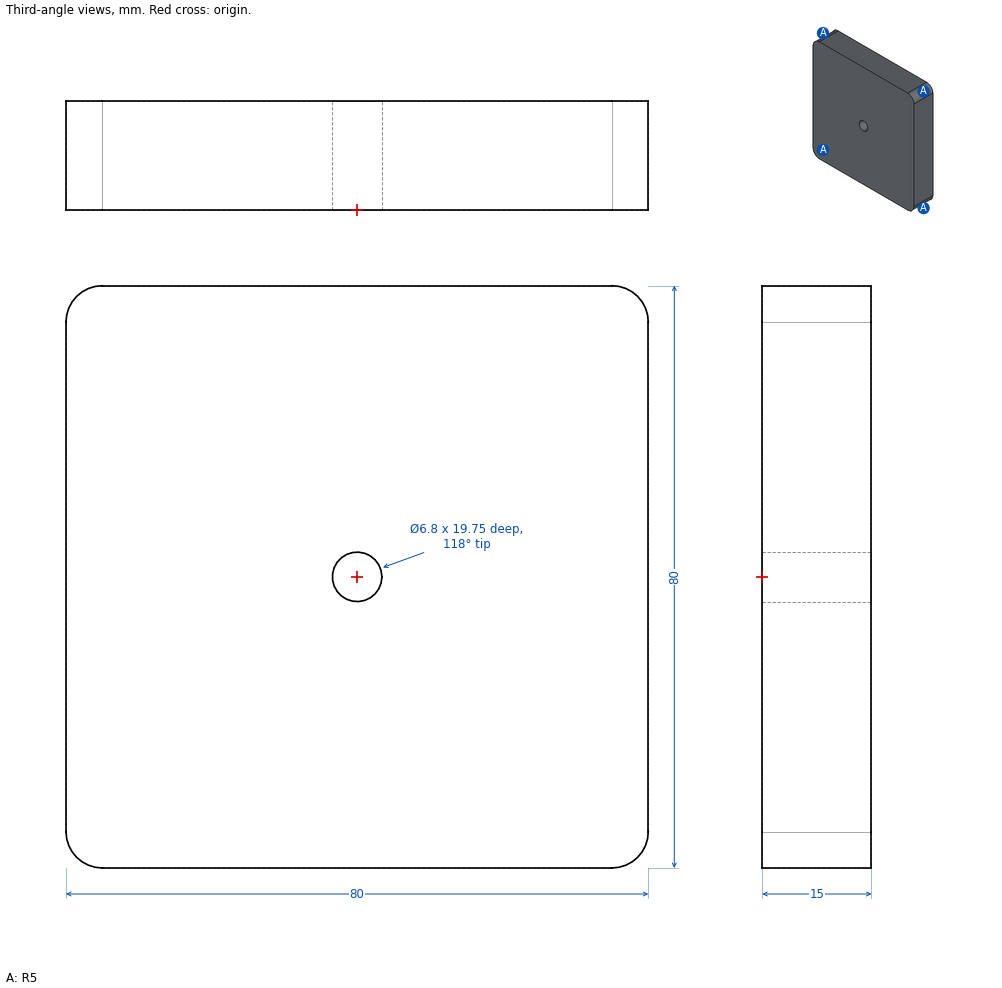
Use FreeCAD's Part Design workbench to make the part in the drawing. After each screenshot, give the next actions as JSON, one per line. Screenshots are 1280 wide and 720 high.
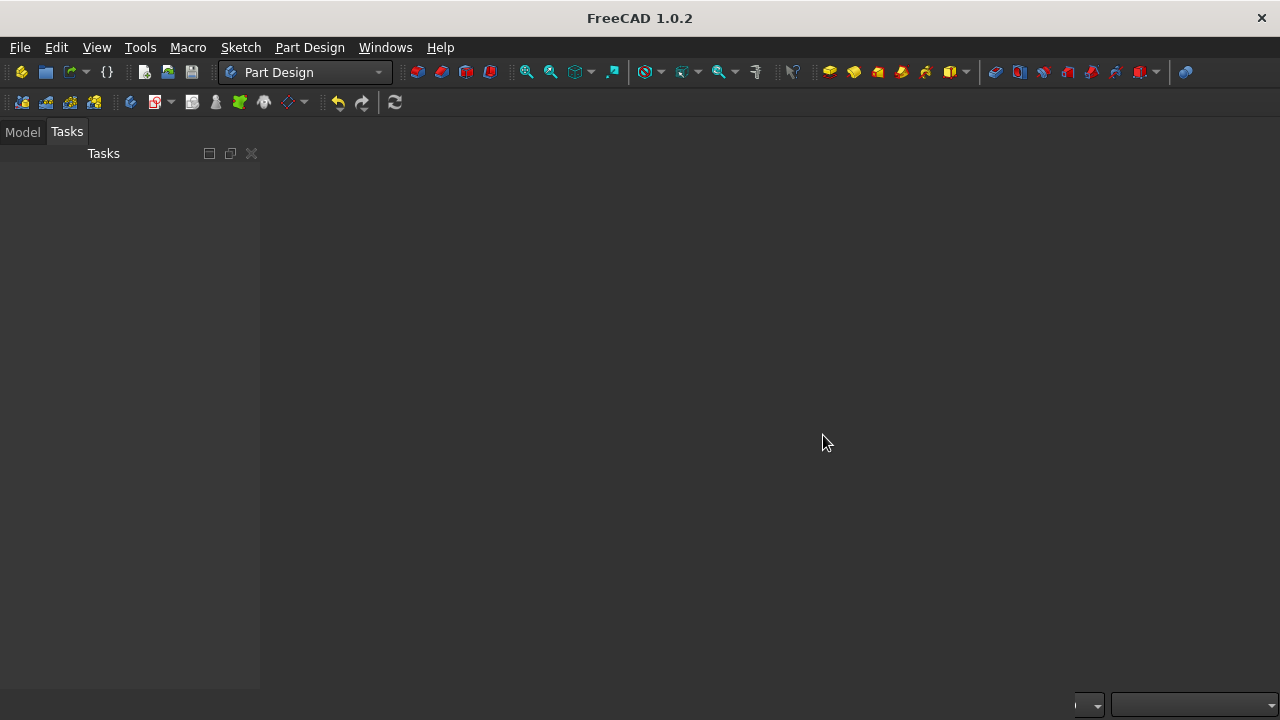
{"action": "key", "text": "ctrl+n"}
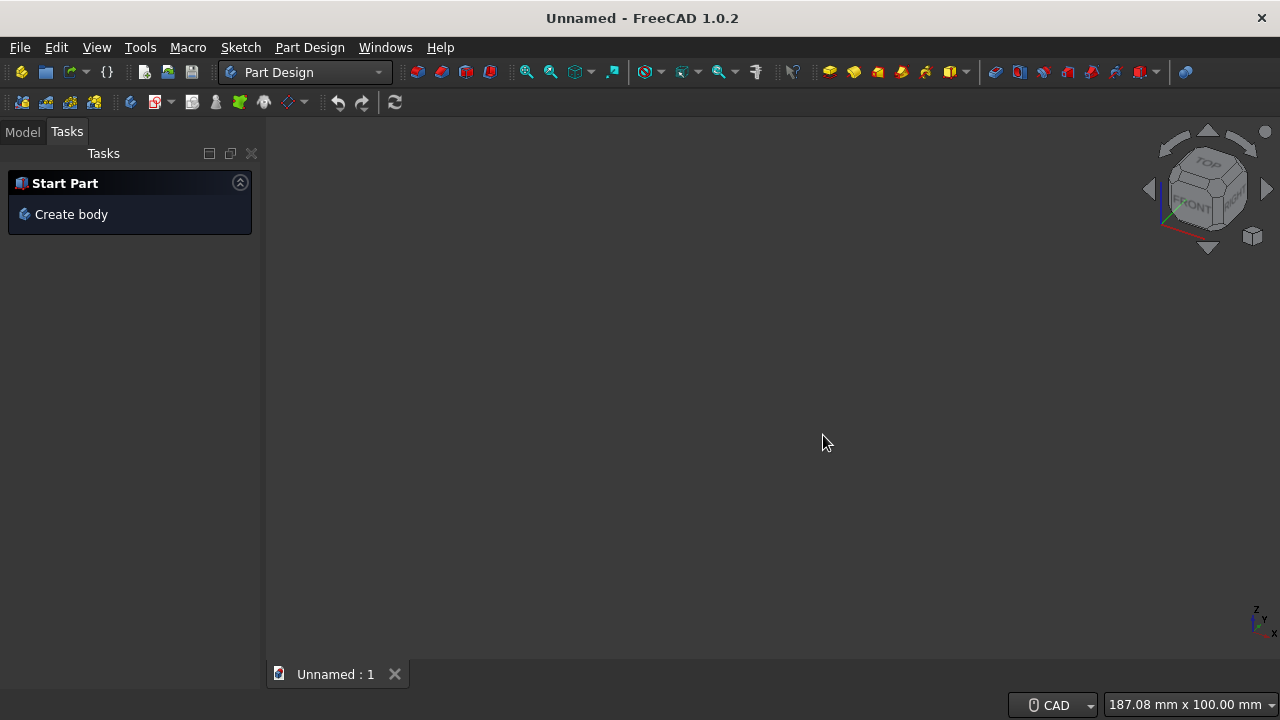
{"action": "left_click", "coordinate": [156, 102]}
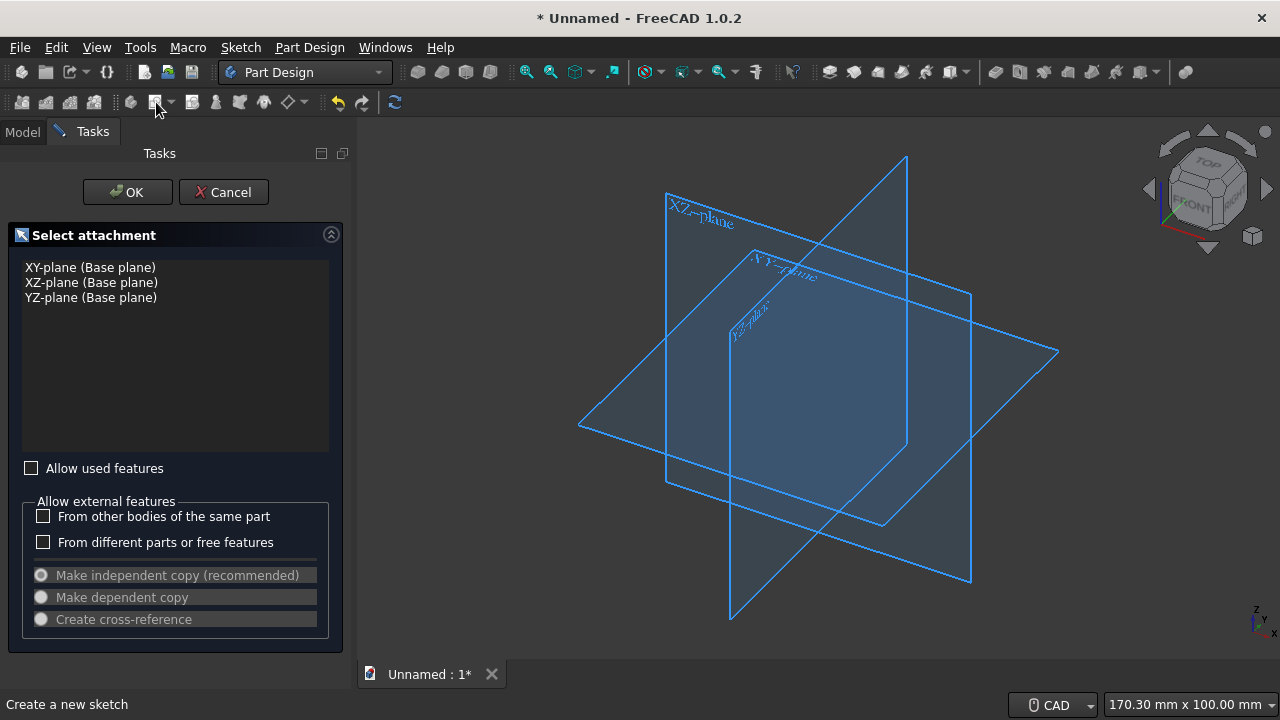
{"action": "left_click", "coordinate": [82, 282]}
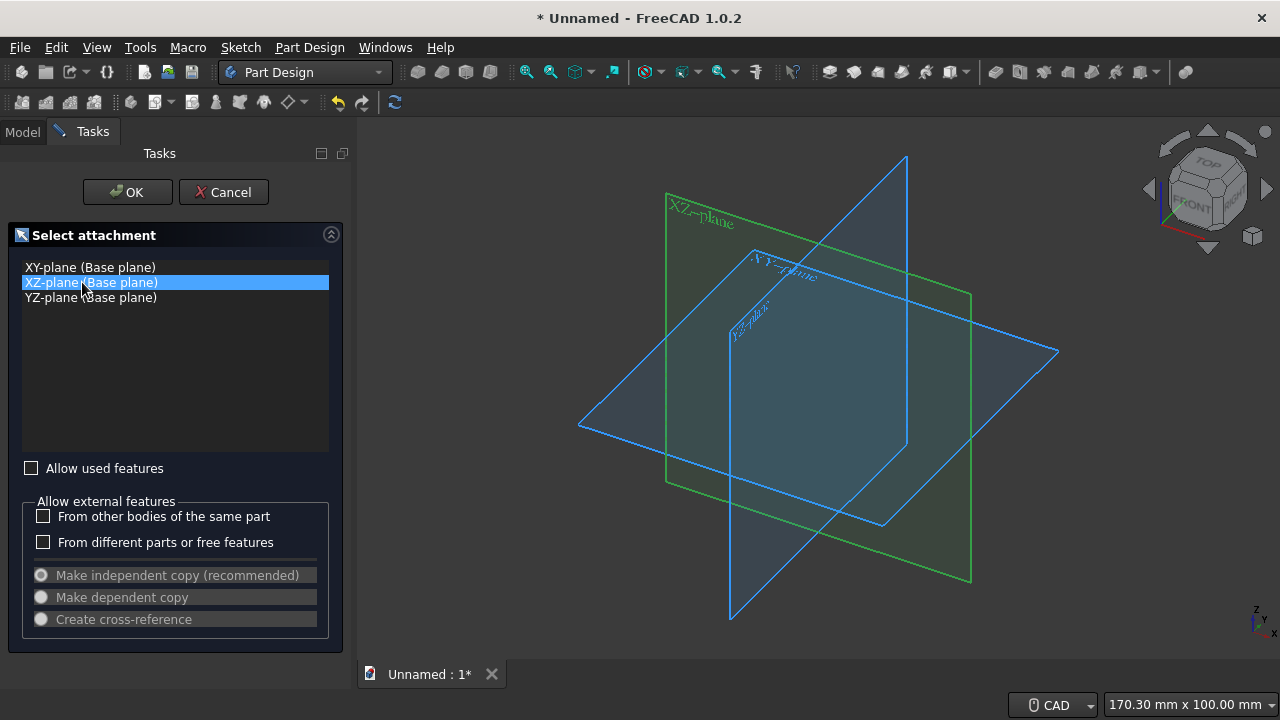
{"action": "left_click", "coordinate": [128, 192]}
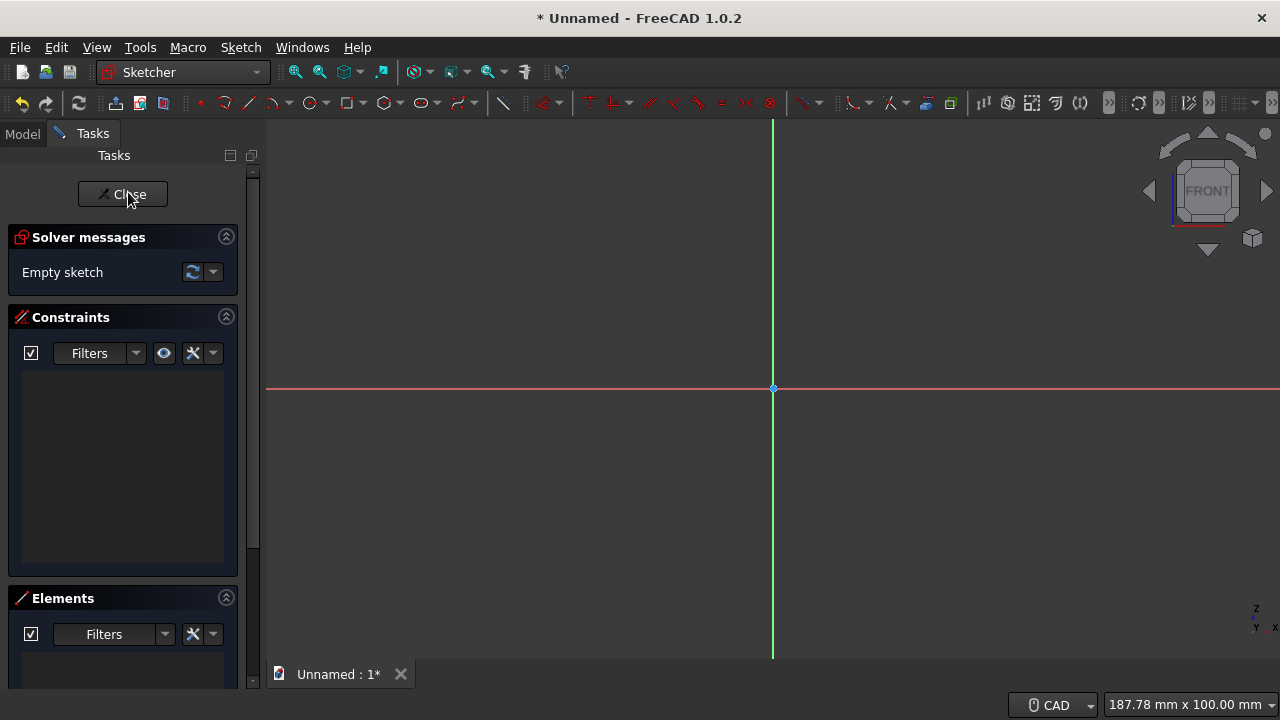
{"action": "key", "text": "g v"}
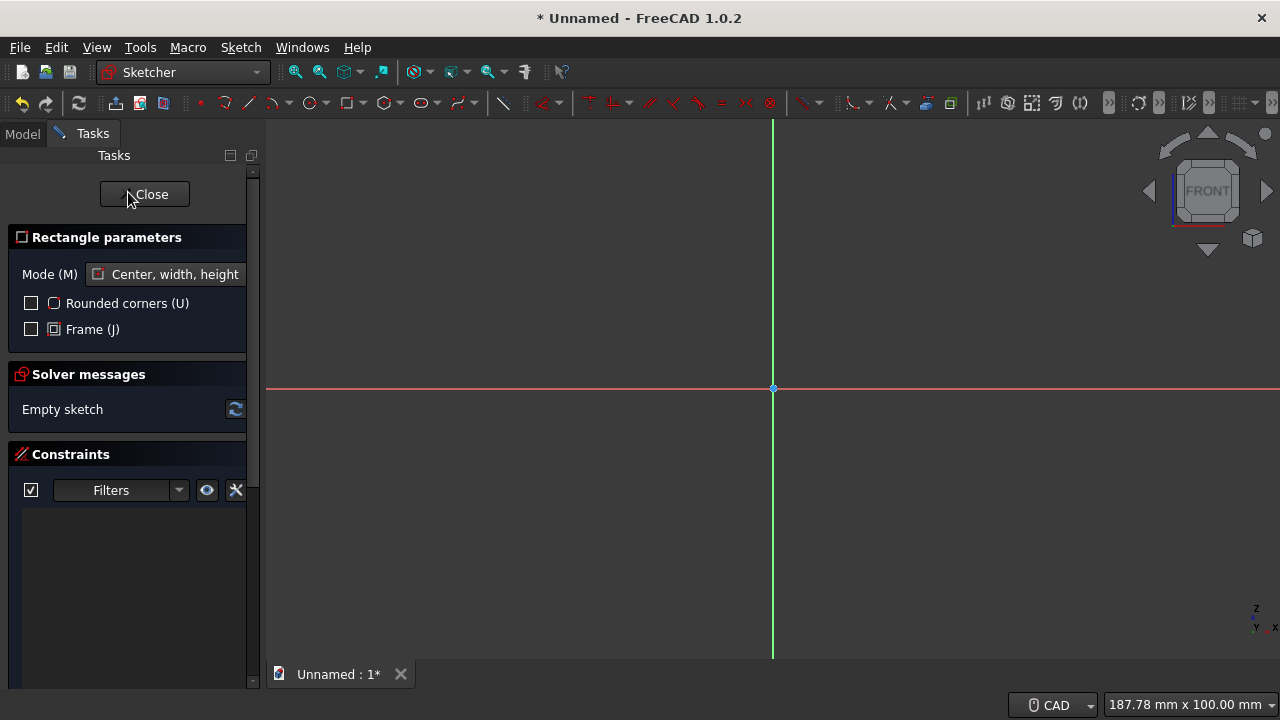
{"action": "left_click", "coordinate": [773, 389]}
{"action": "mouse_move", "coordinate": [989, 173]}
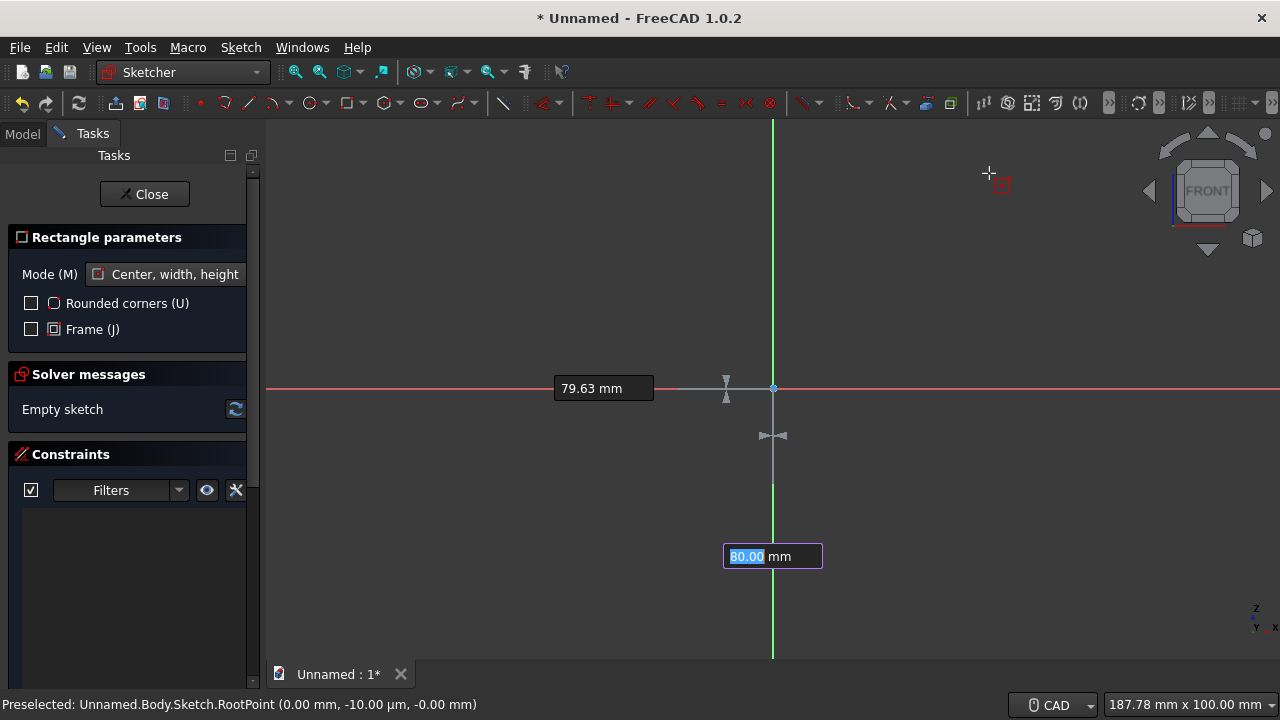
{"action": "type", "text": "80"}
{"action": "key", "text": "Tab"}
{"action": "type", "text": "80"}
{"action": "key", "text": "Return"}
{"action": "key", "text": "Escape"}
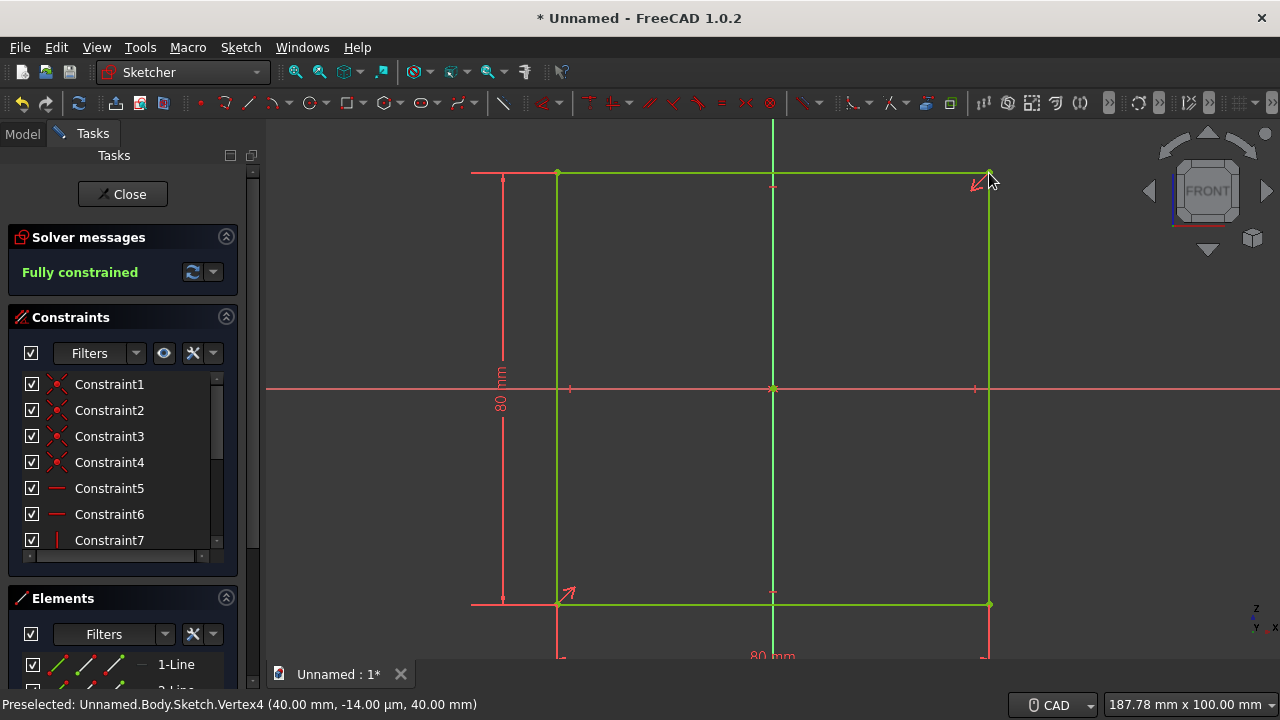
{"action": "left_click", "coordinate": [123, 194]}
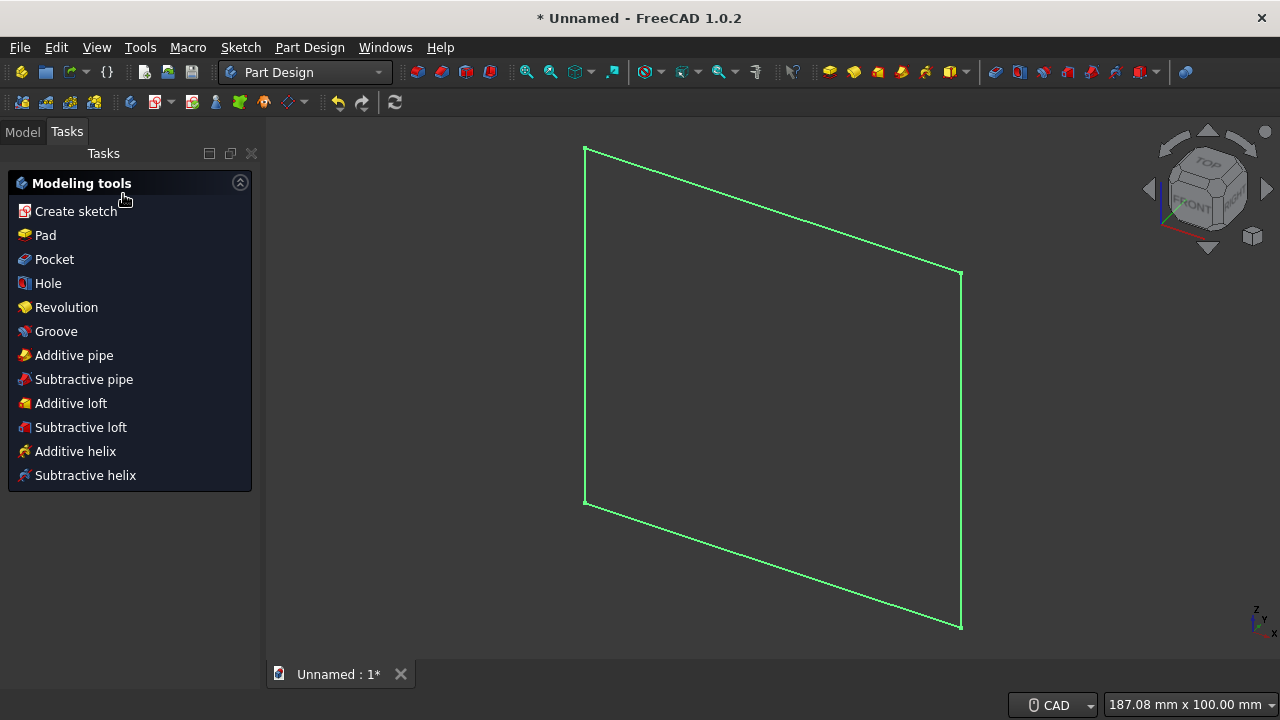
{"action": "left_click", "coordinate": [830, 72]}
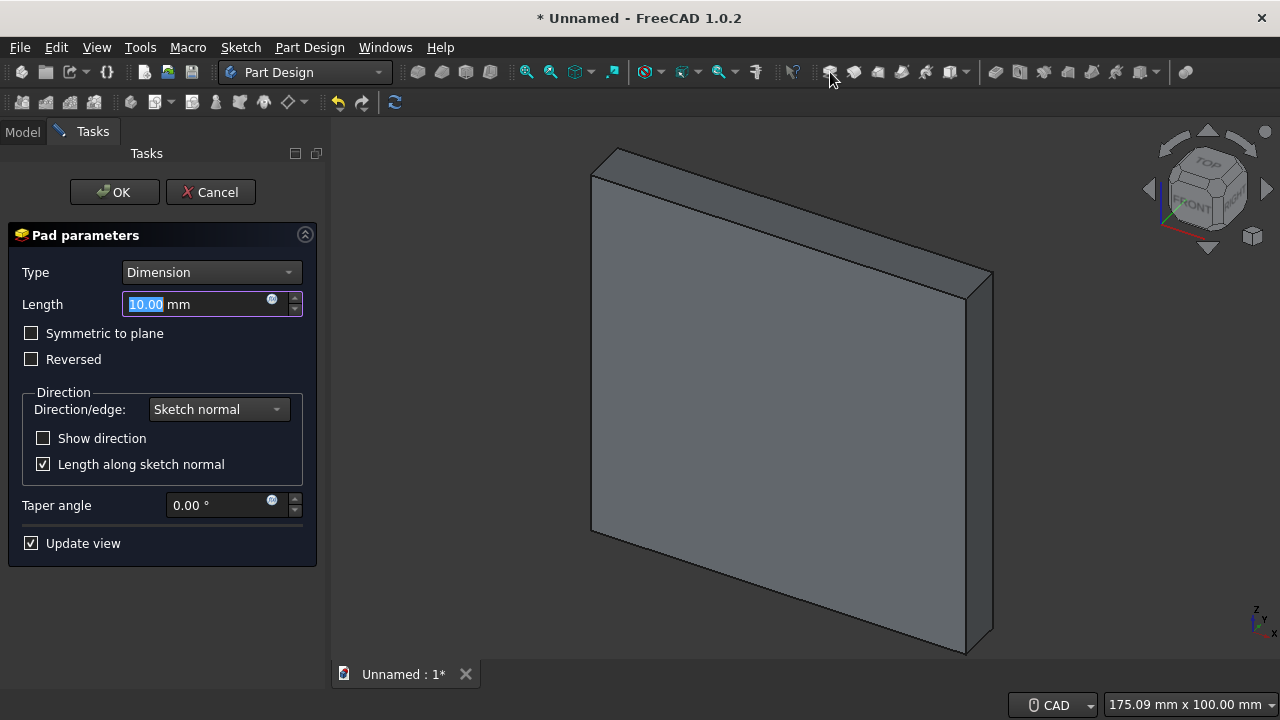
{"action": "type", "text": "15"}
{"action": "key", "text": "Tab"}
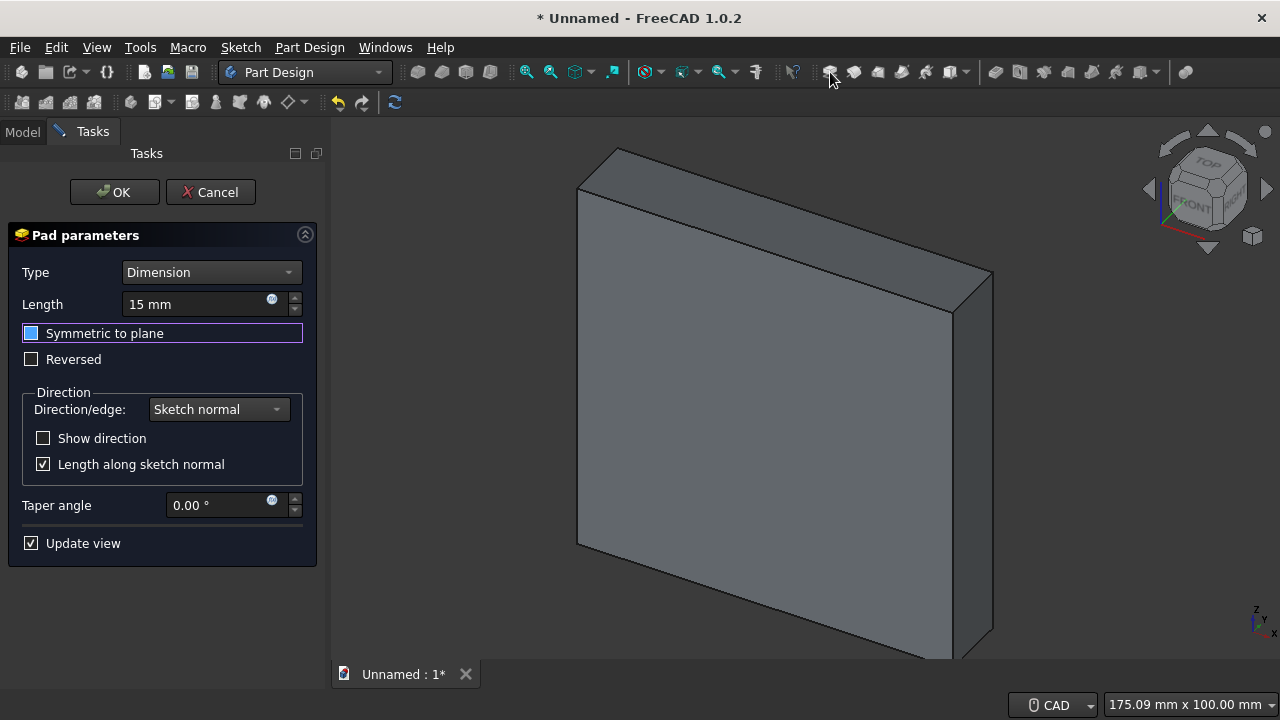
{"action": "left_click", "coordinate": [30, 359]}